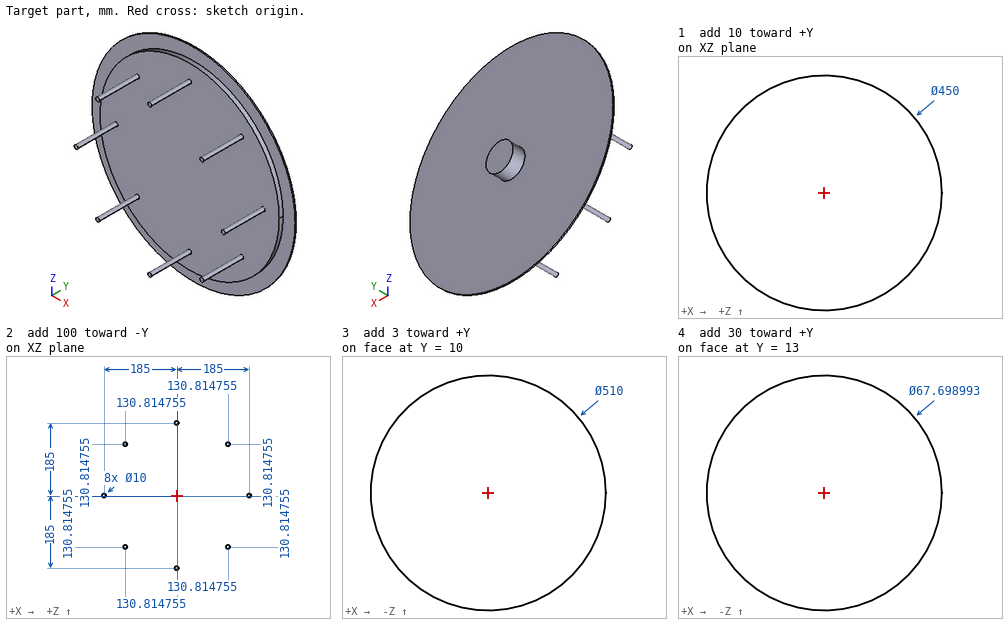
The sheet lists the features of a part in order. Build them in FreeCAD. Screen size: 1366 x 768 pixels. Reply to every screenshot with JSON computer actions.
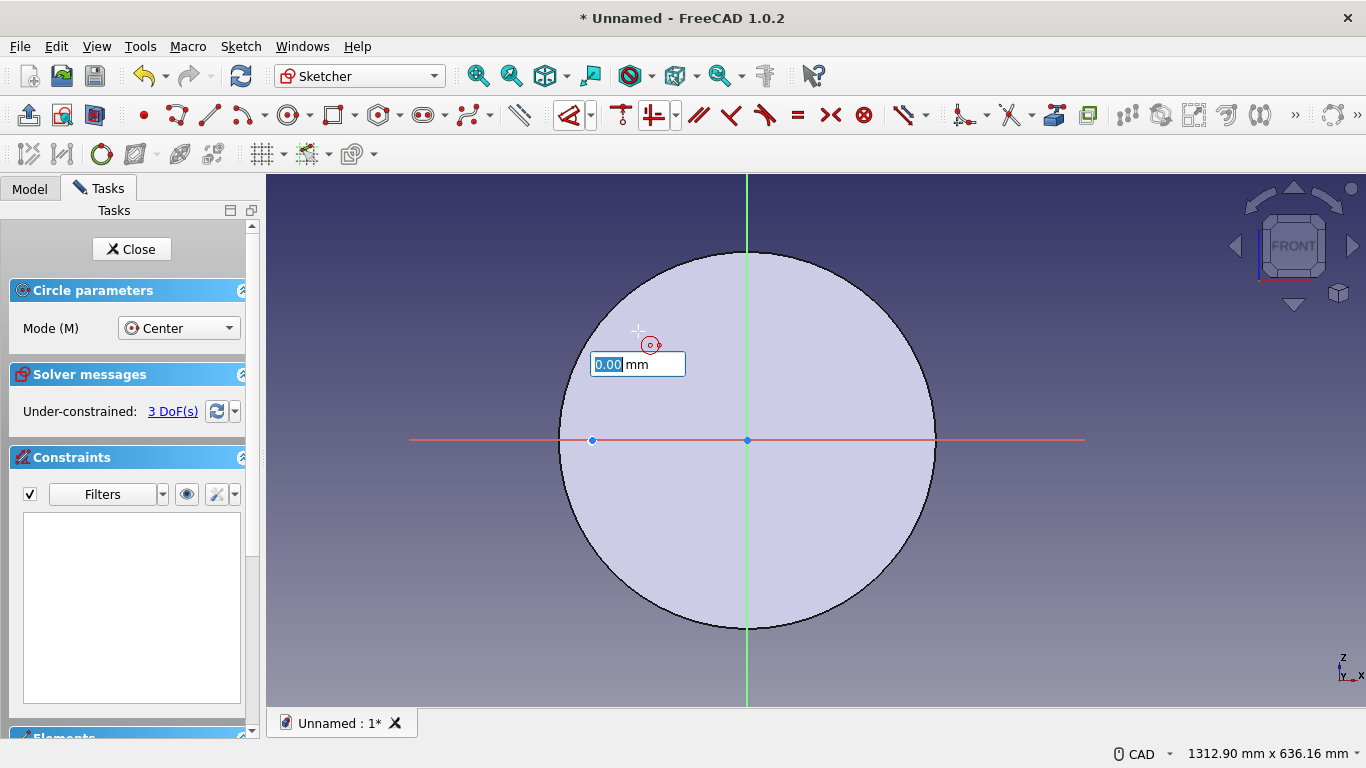
{"action": "scroll", "coordinate": [641, 328], "scroll_direction": "up", "scroll_amount": 7}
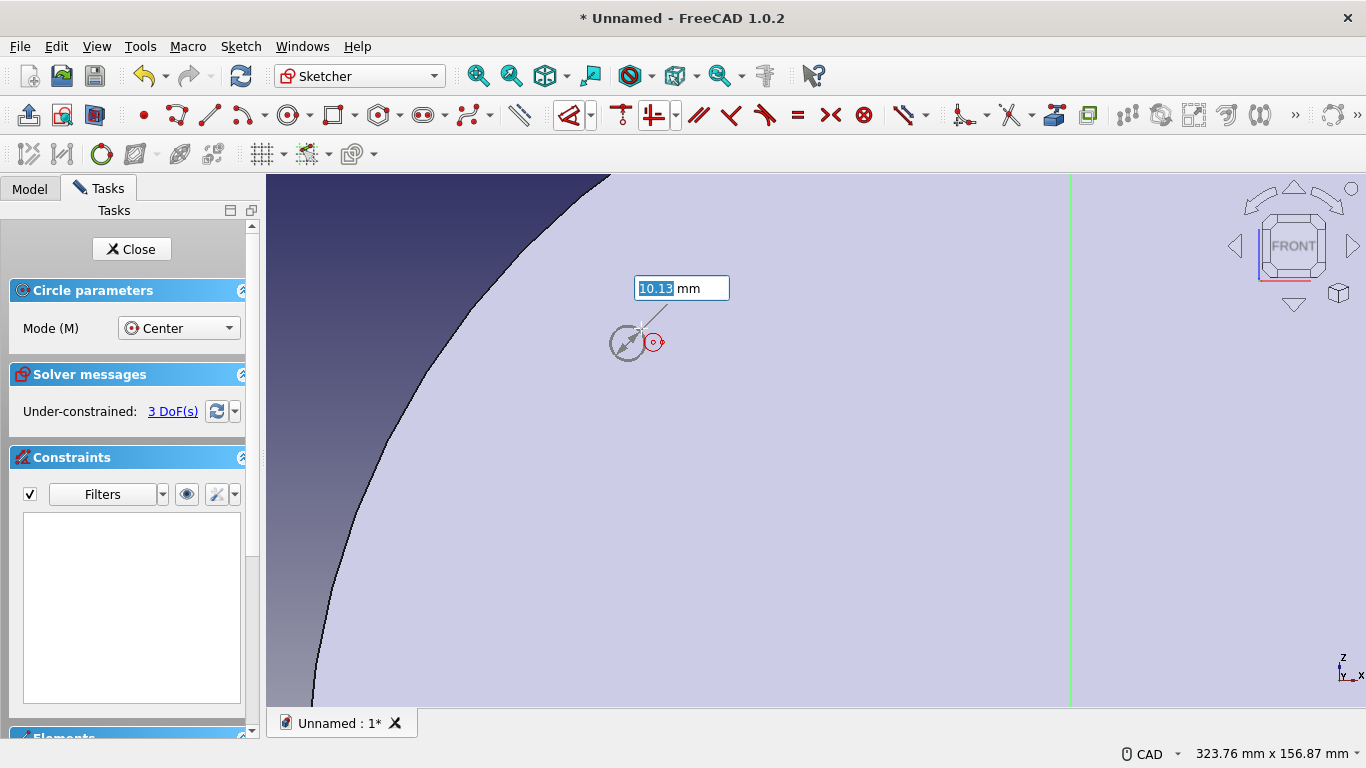
{"action": "left_click", "coordinate": [639, 327]}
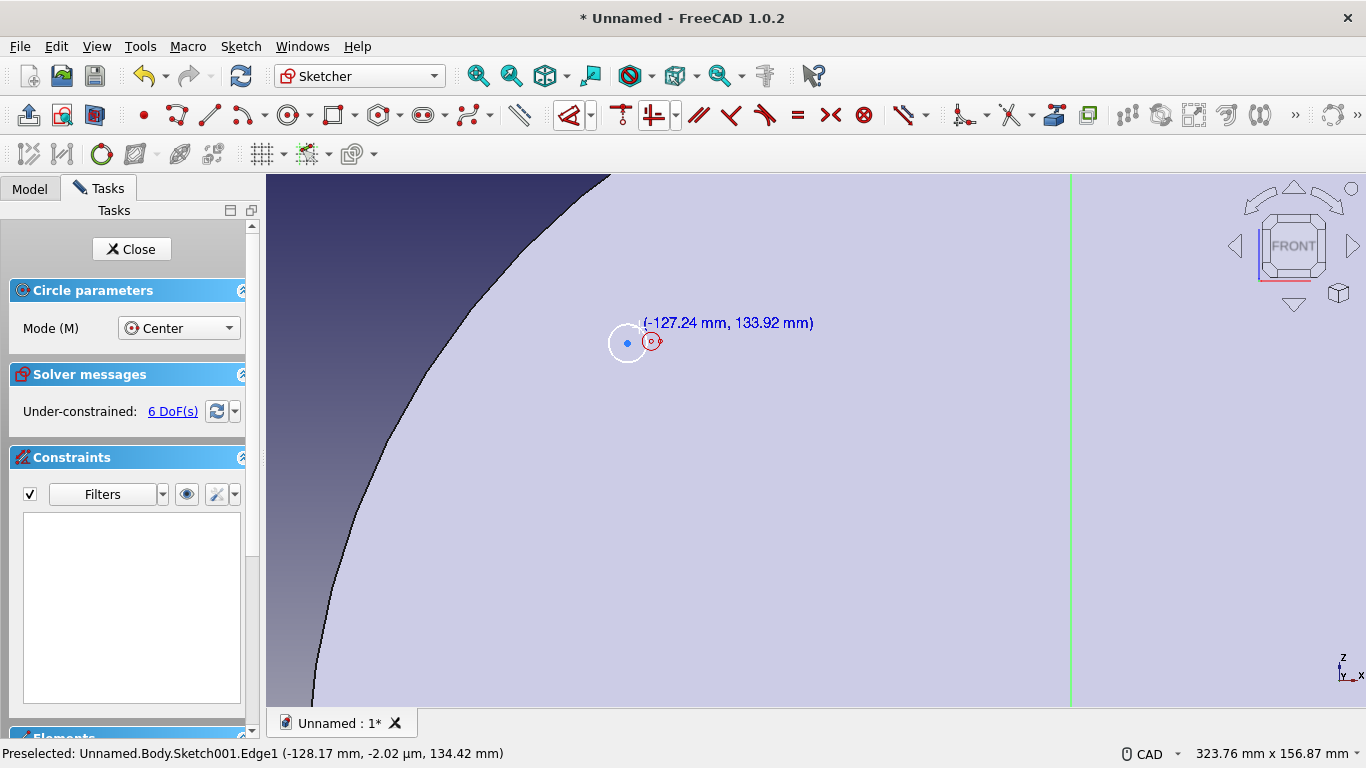
{"action": "scroll", "coordinate": [642, 328], "scroll_direction": "down", "scroll_amount": 7}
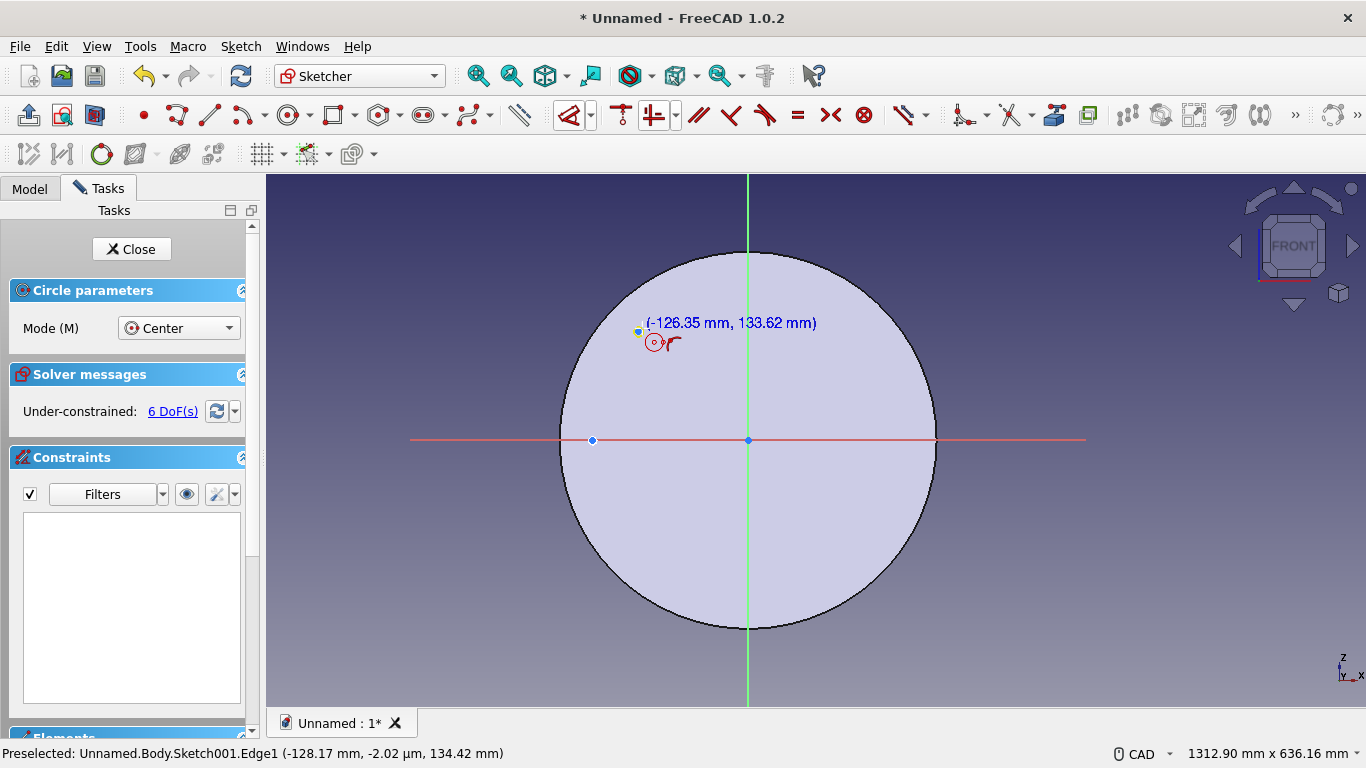
{"action": "scroll", "coordinate": [748, 285], "scroll_direction": "up", "scroll_amount": 9}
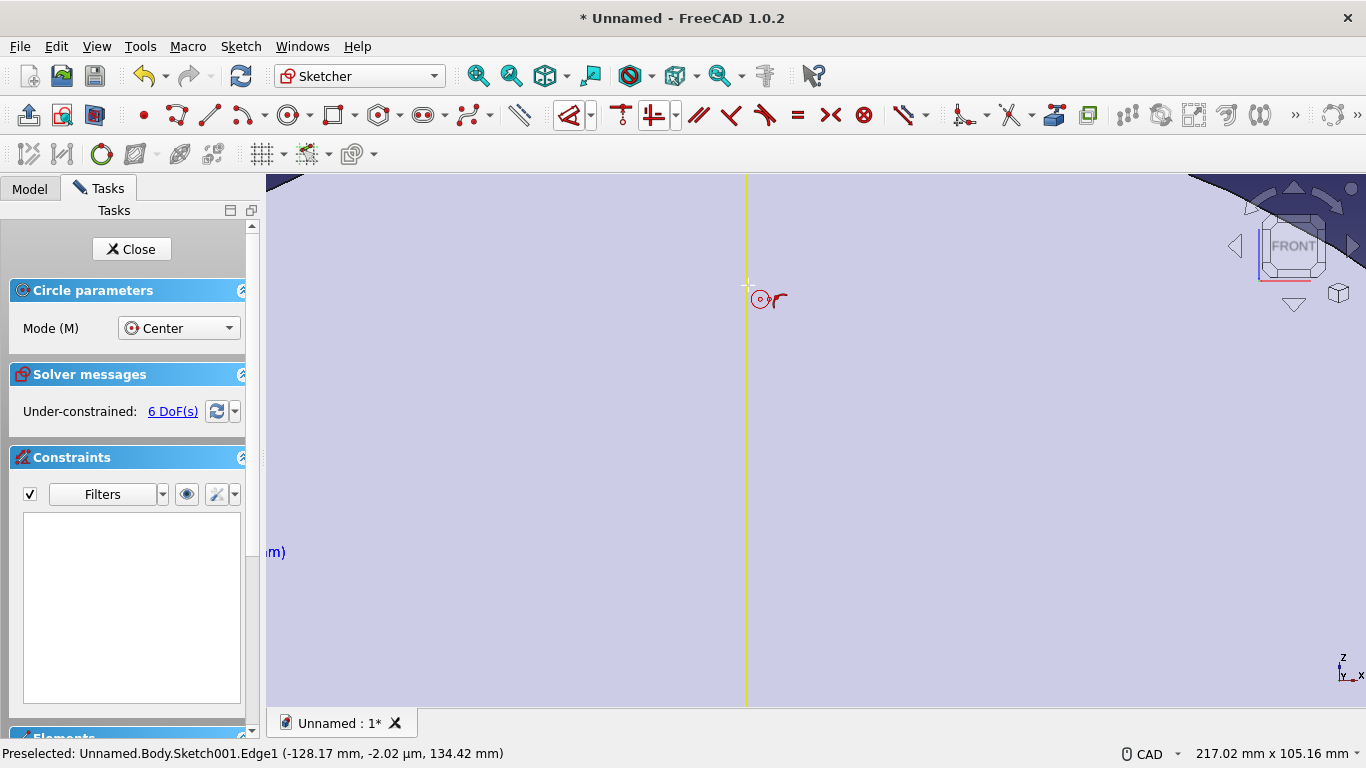
{"action": "scroll", "coordinate": [748, 285], "scroll_direction": "down", "scroll_amount": 9}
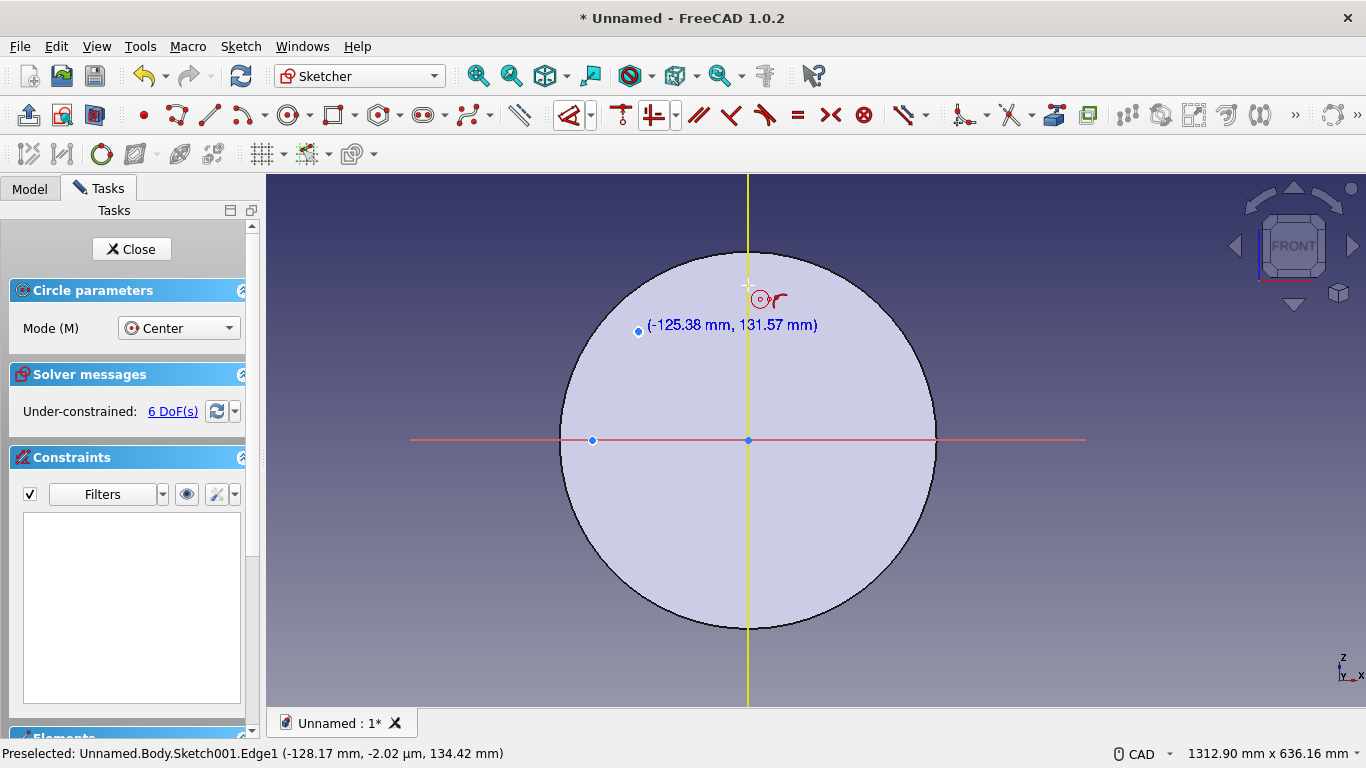
{"action": "left_click", "coordinate": [748, 285]}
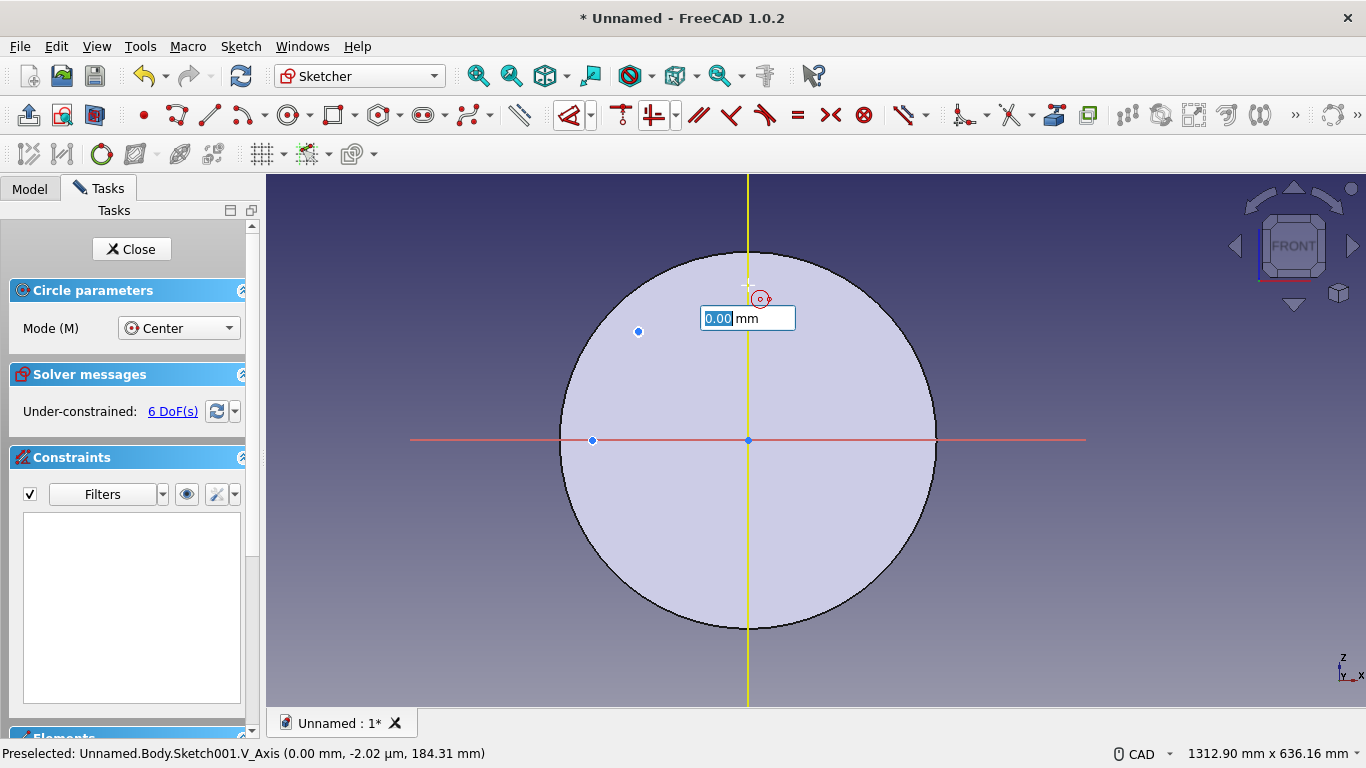
{"action": "scroll", "coordinate": [752, 284], "scroll_direction": "up", "scroll_amount": 7}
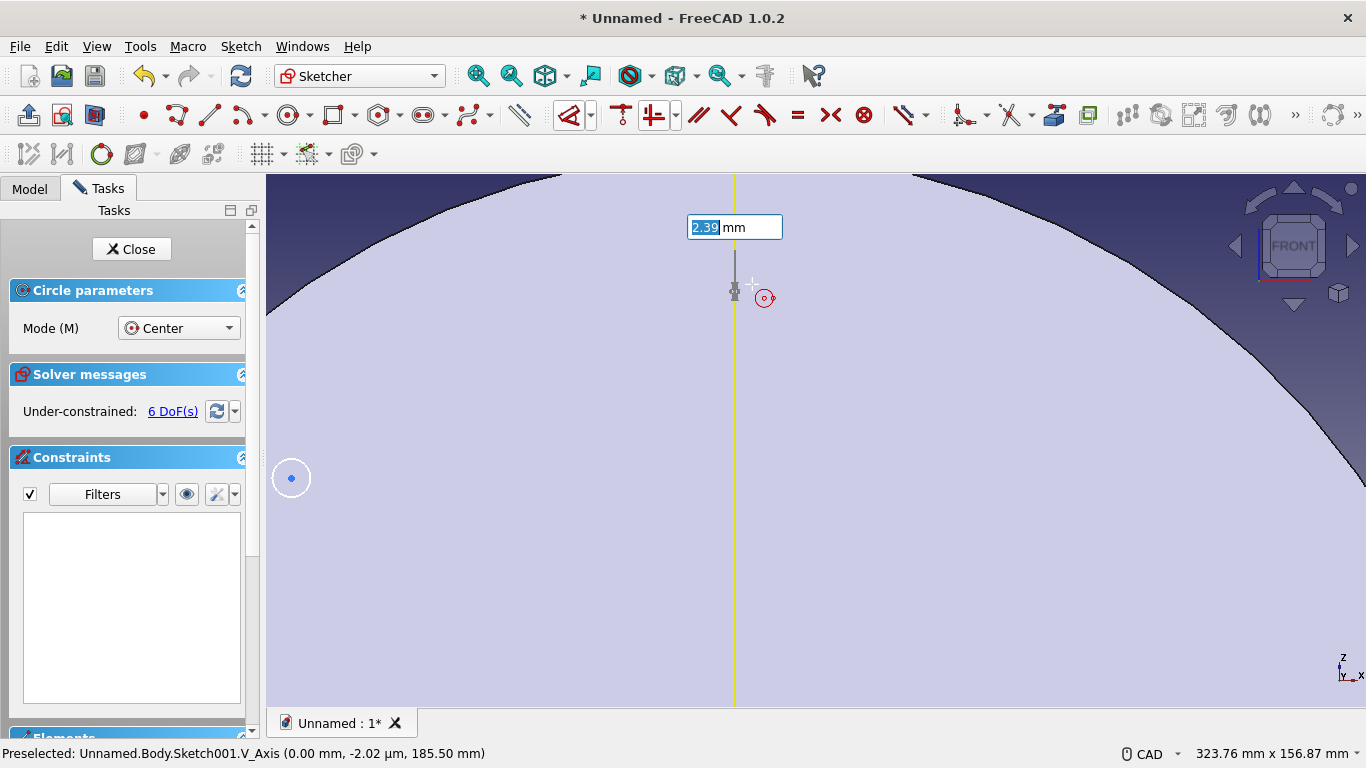
{"action": "left_click", "coordinate": [751, 283]}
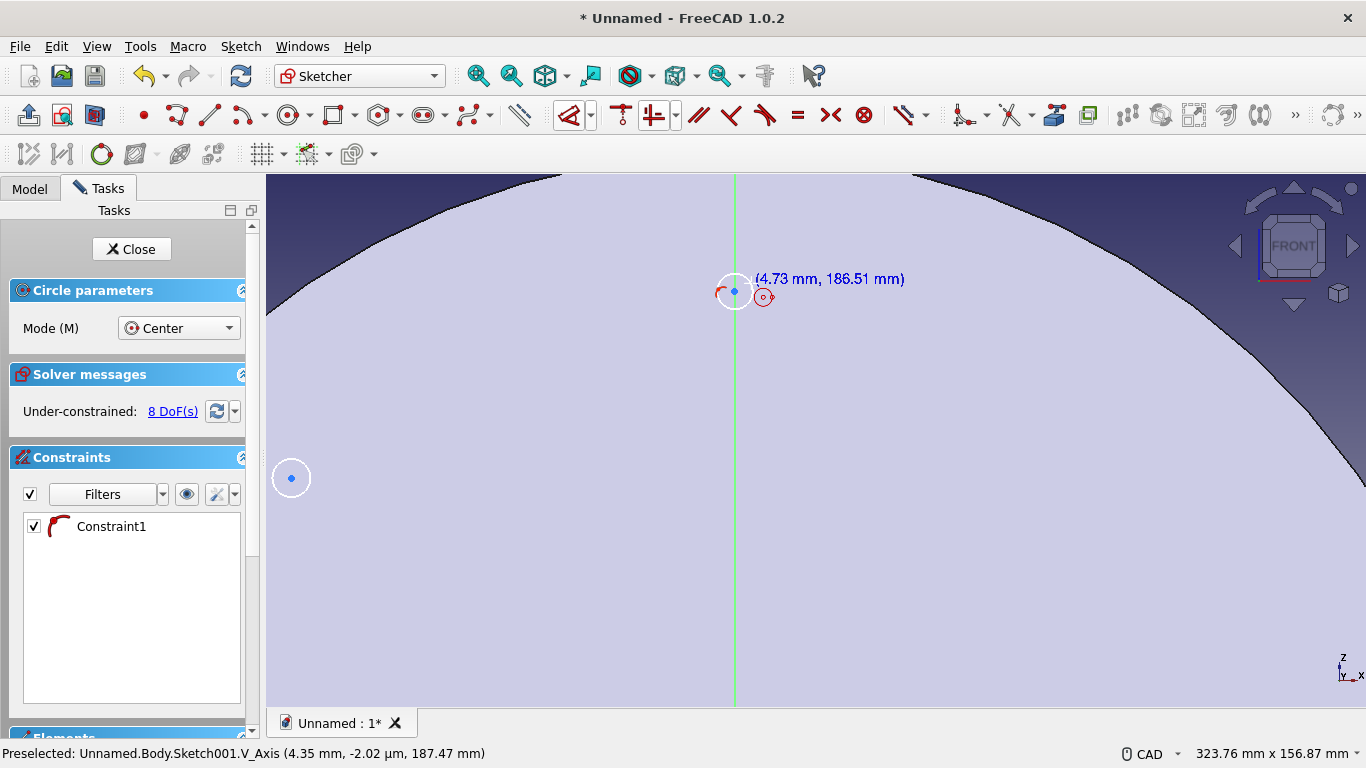
{"action": "scroll", "coordinate": [1179, 473], "scroll_direction": "up", "scroll_amount": 2}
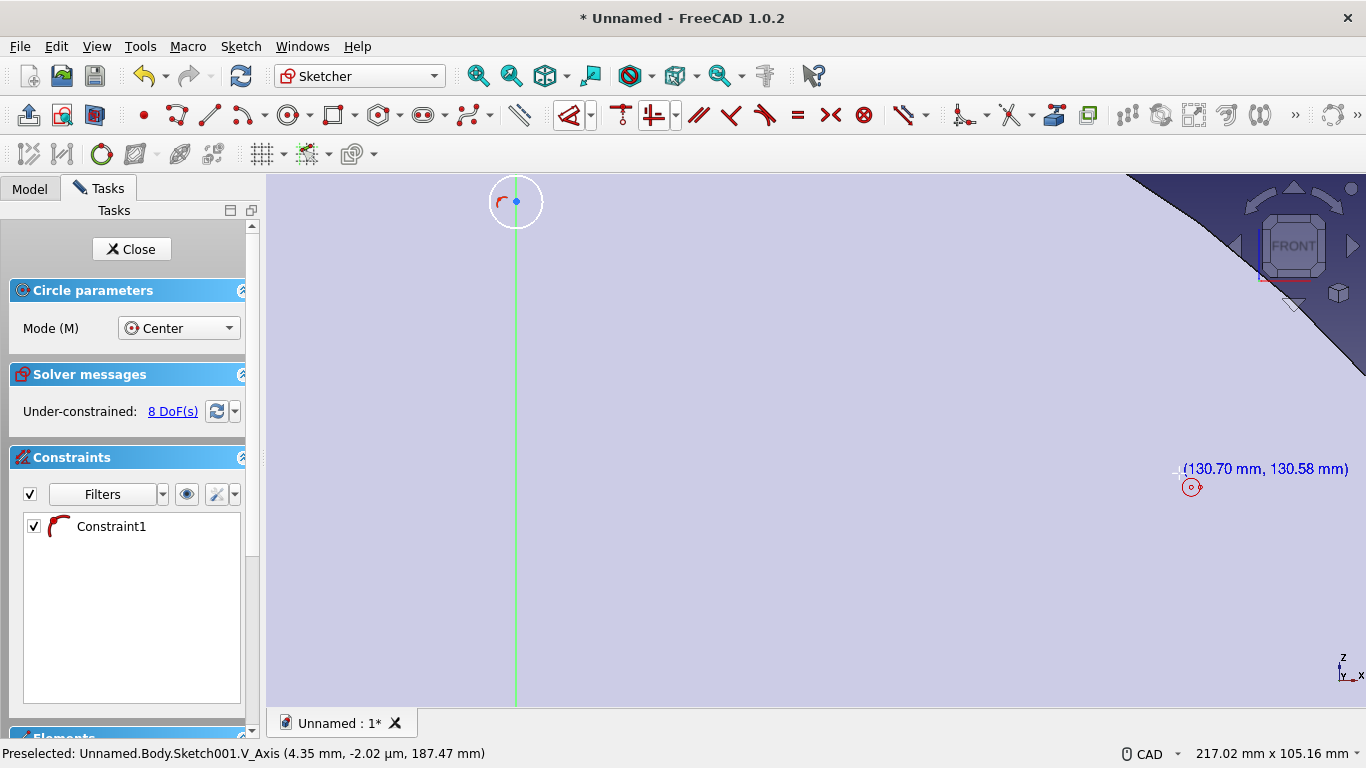
{"action": "scroll", "coordinate": [793, 303], "scroll_direction": "down", "scroll_amount": 9}